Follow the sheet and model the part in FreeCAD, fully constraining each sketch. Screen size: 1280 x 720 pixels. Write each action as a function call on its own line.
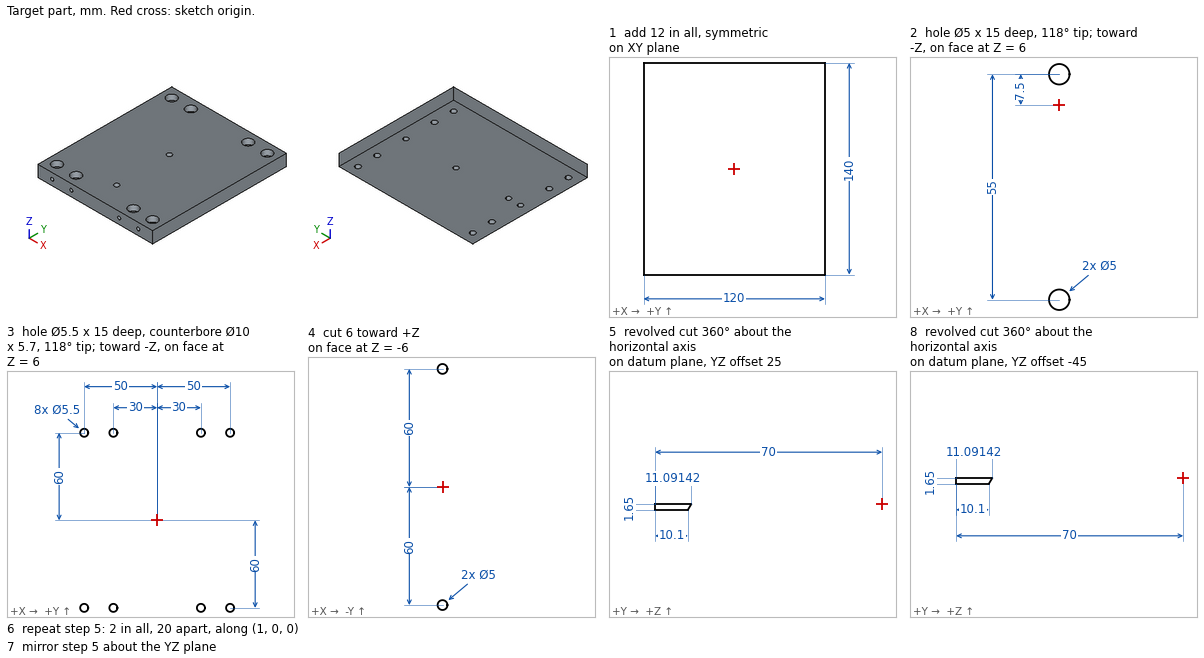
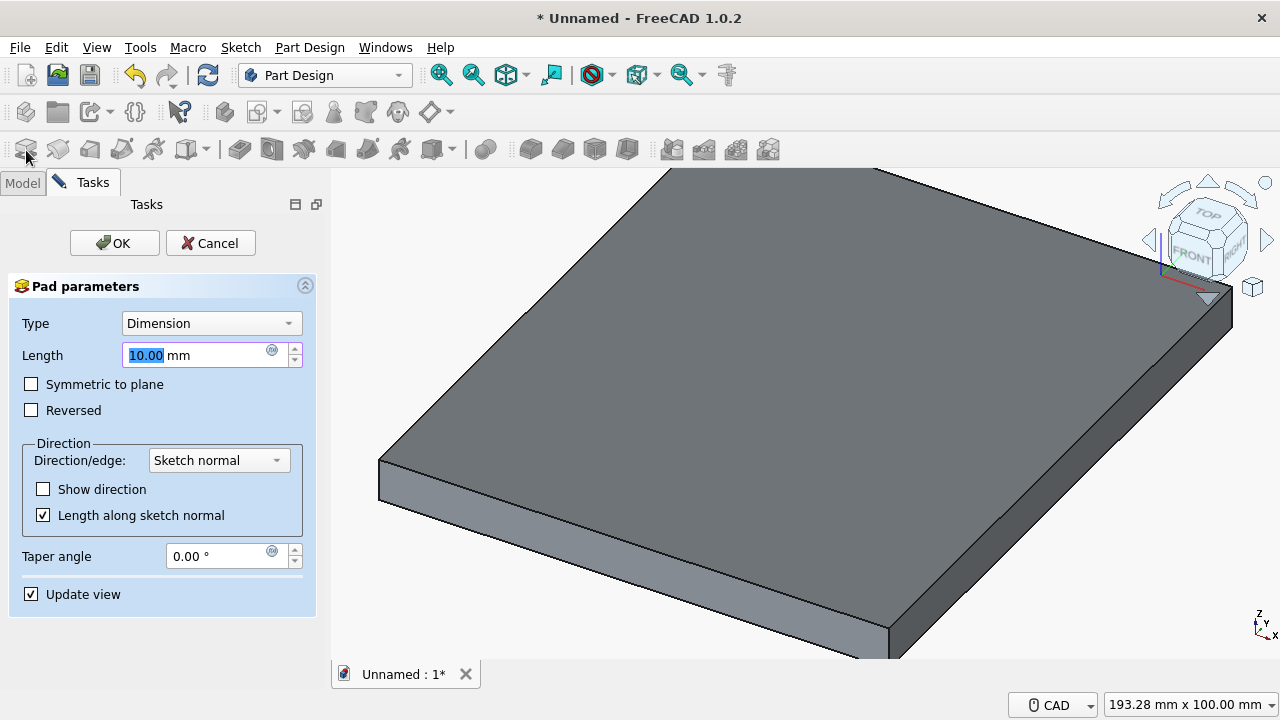
text(12)
key(Tab)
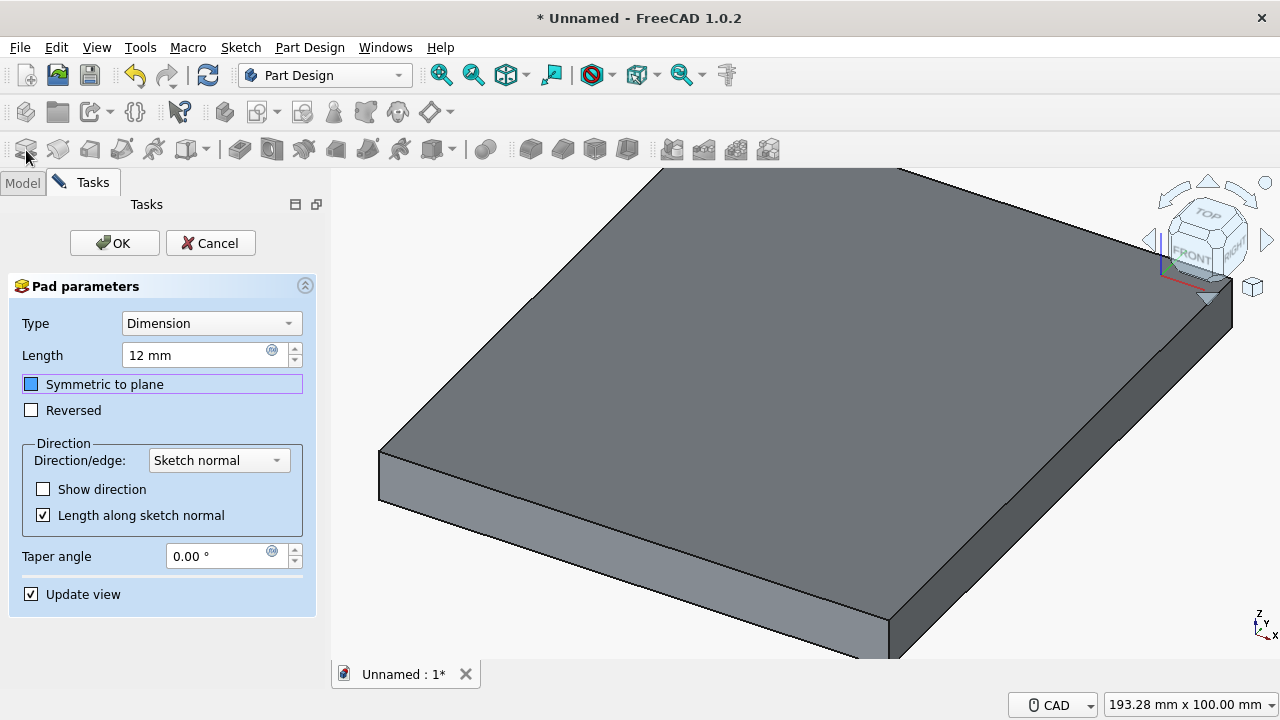
click(30, 384)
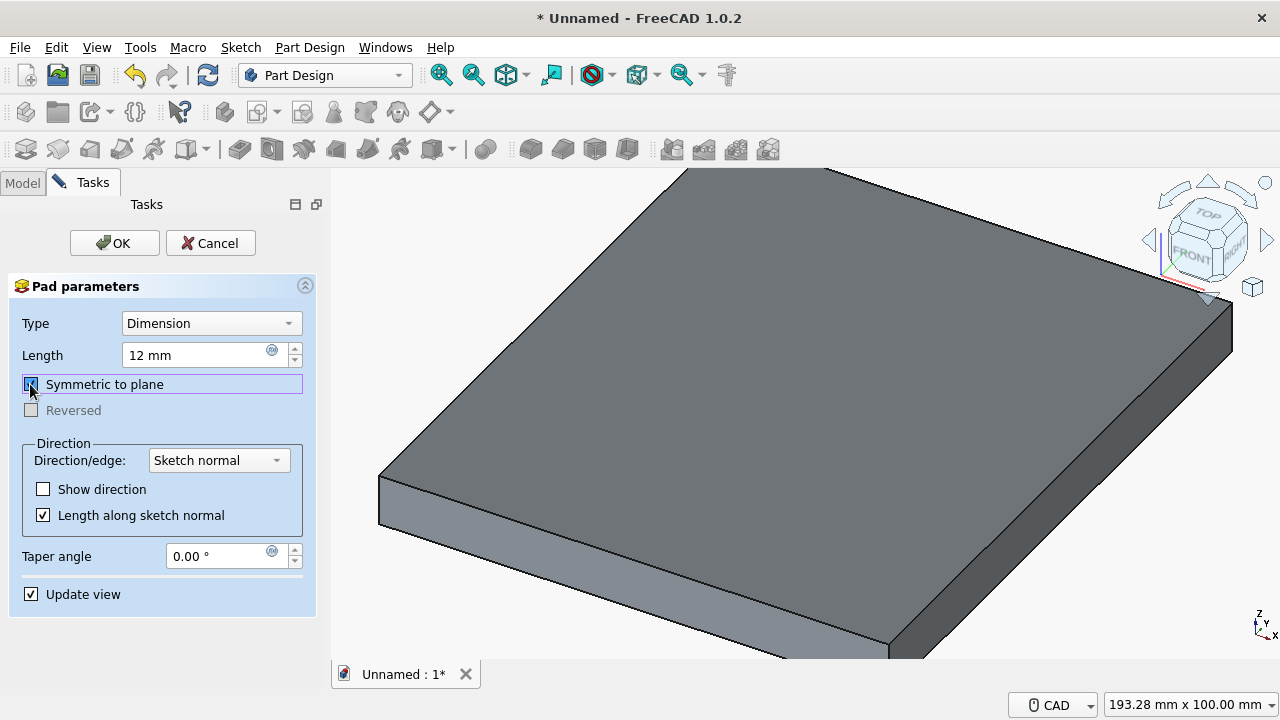
click(115, 243)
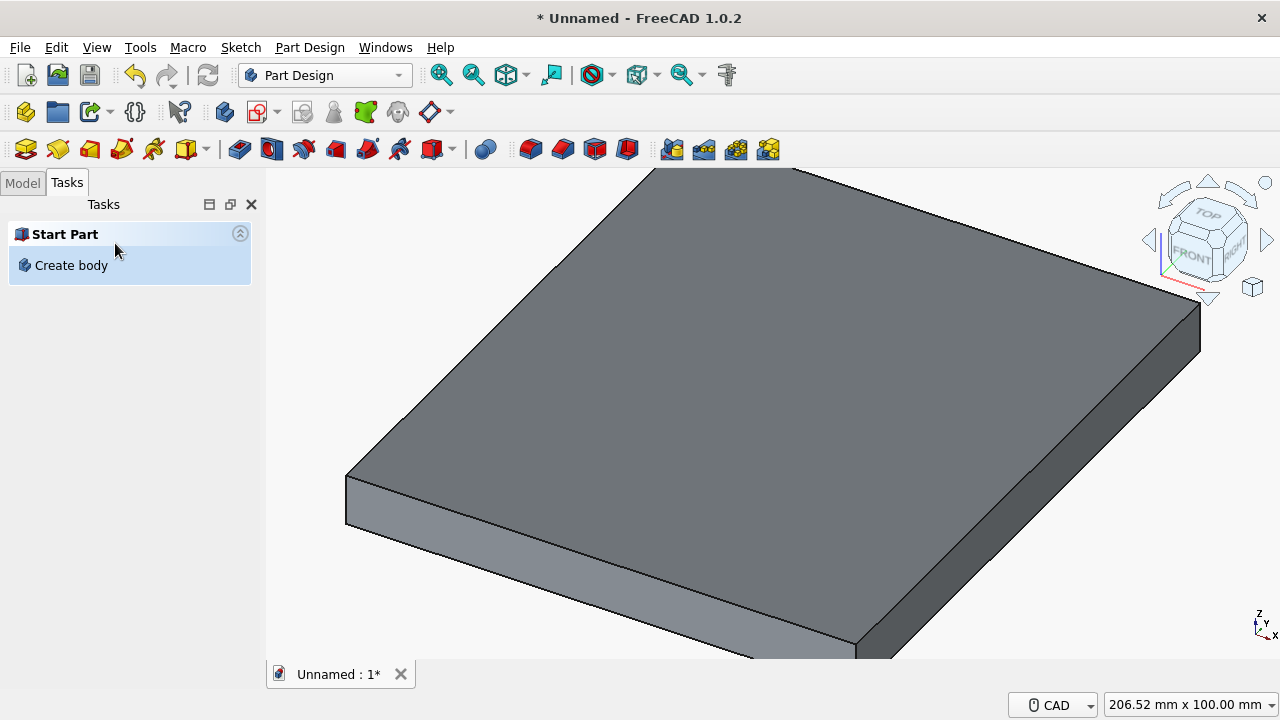
click(442, 76)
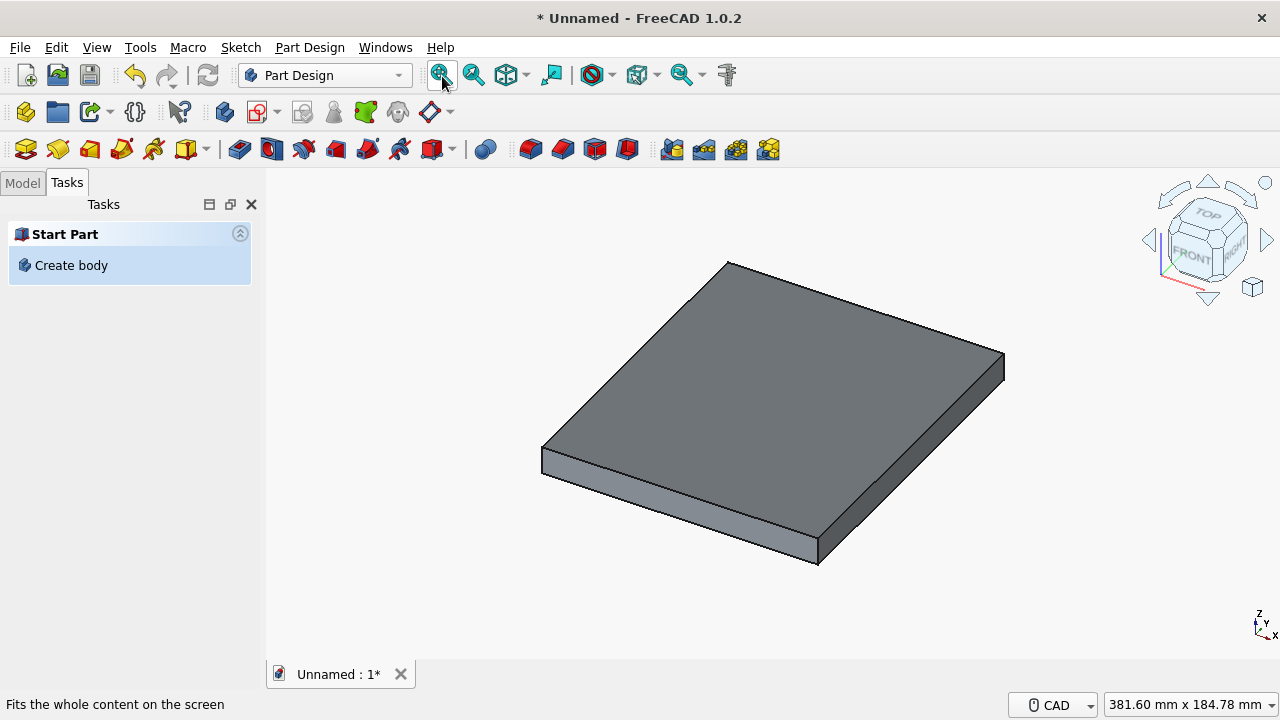
click(773, 399)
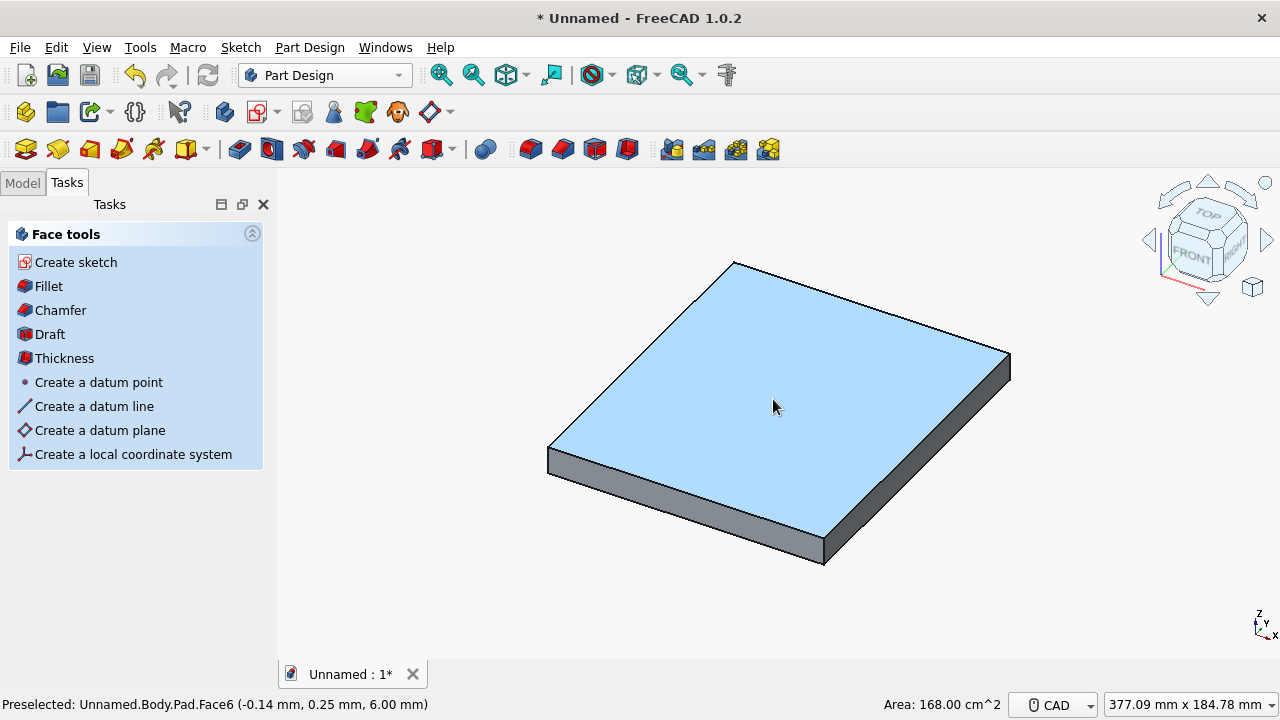
click(258, 112)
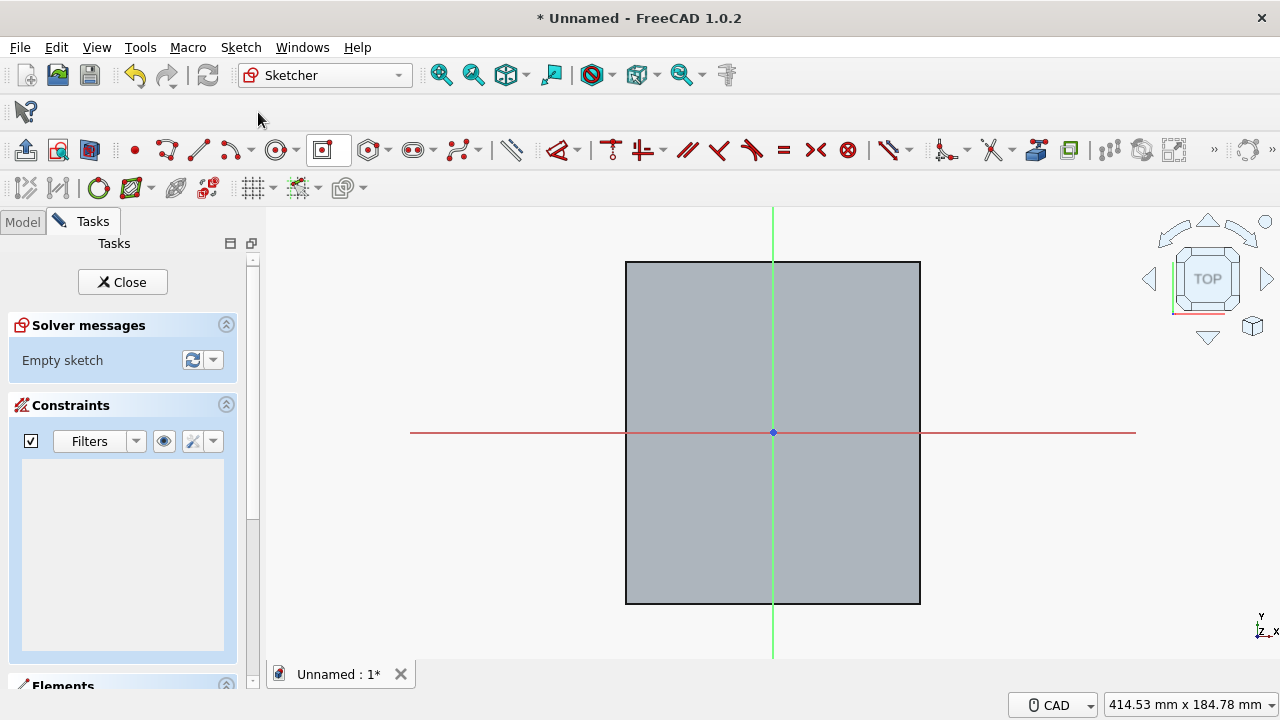
scroll(856, 541, up, 3)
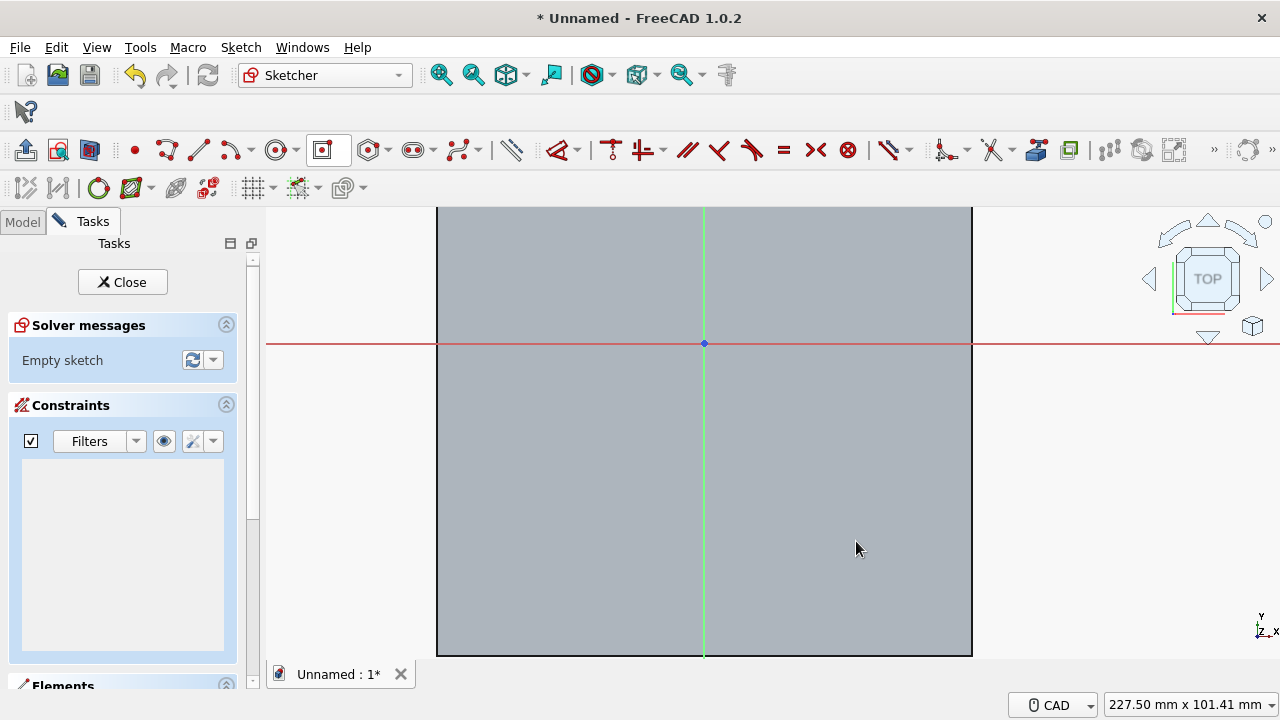
key(g)
key(c)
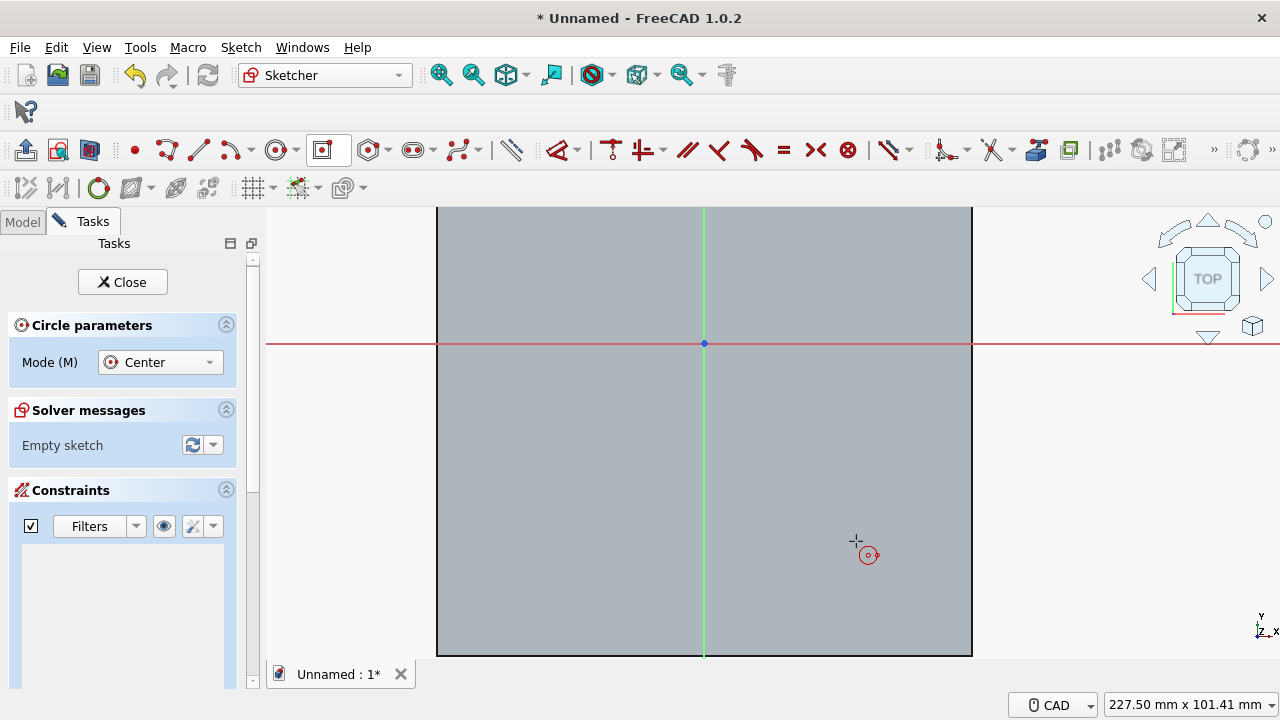
scroll(704, 555, up, 4)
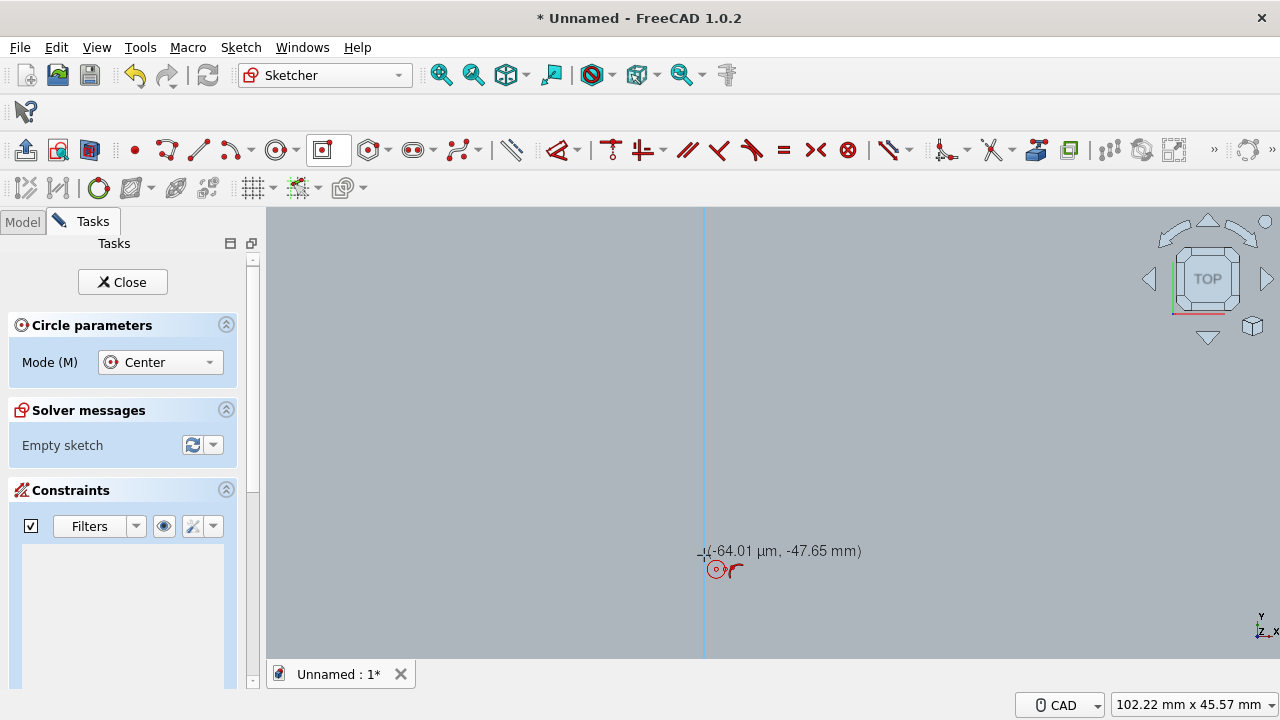
click(704, 555)
move(722, 537)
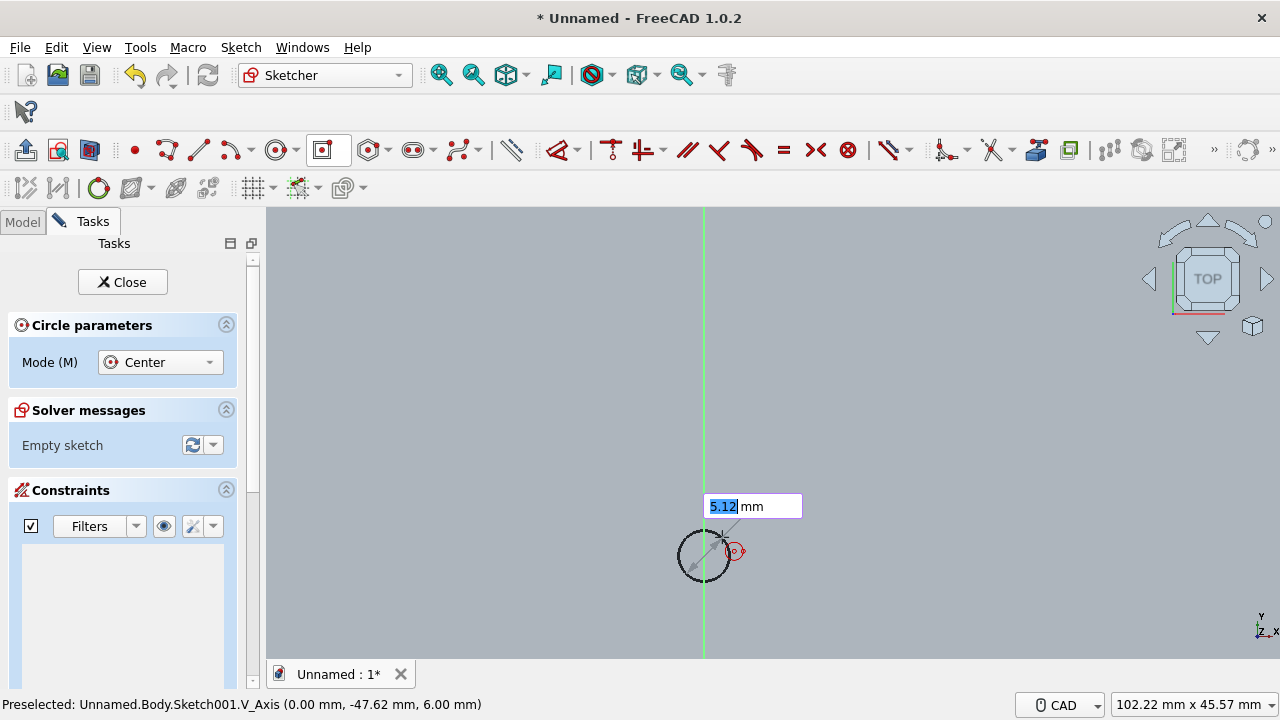
text(5)
key(Return)